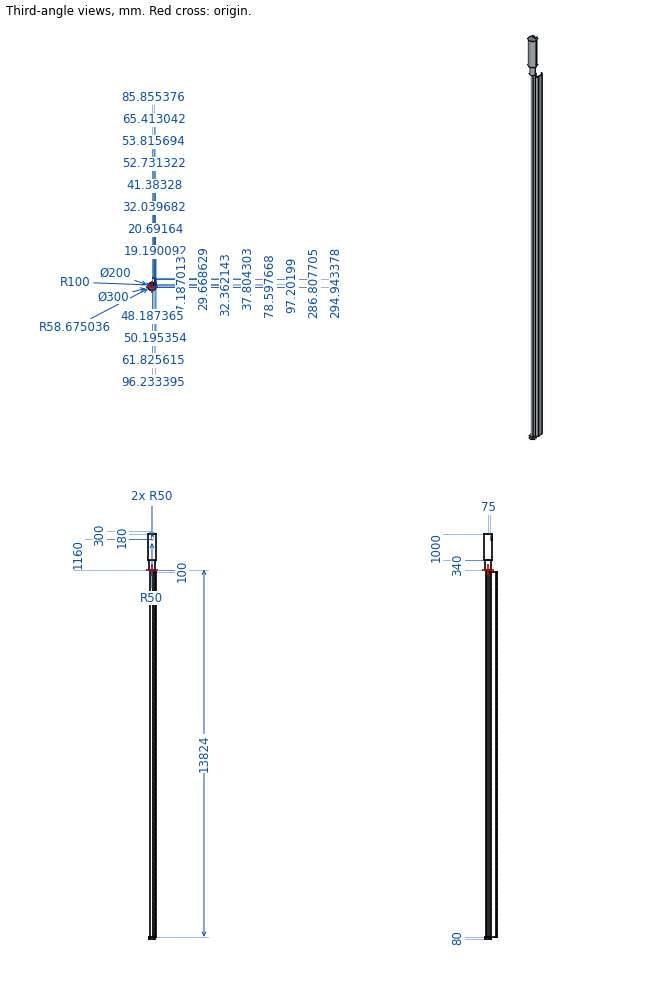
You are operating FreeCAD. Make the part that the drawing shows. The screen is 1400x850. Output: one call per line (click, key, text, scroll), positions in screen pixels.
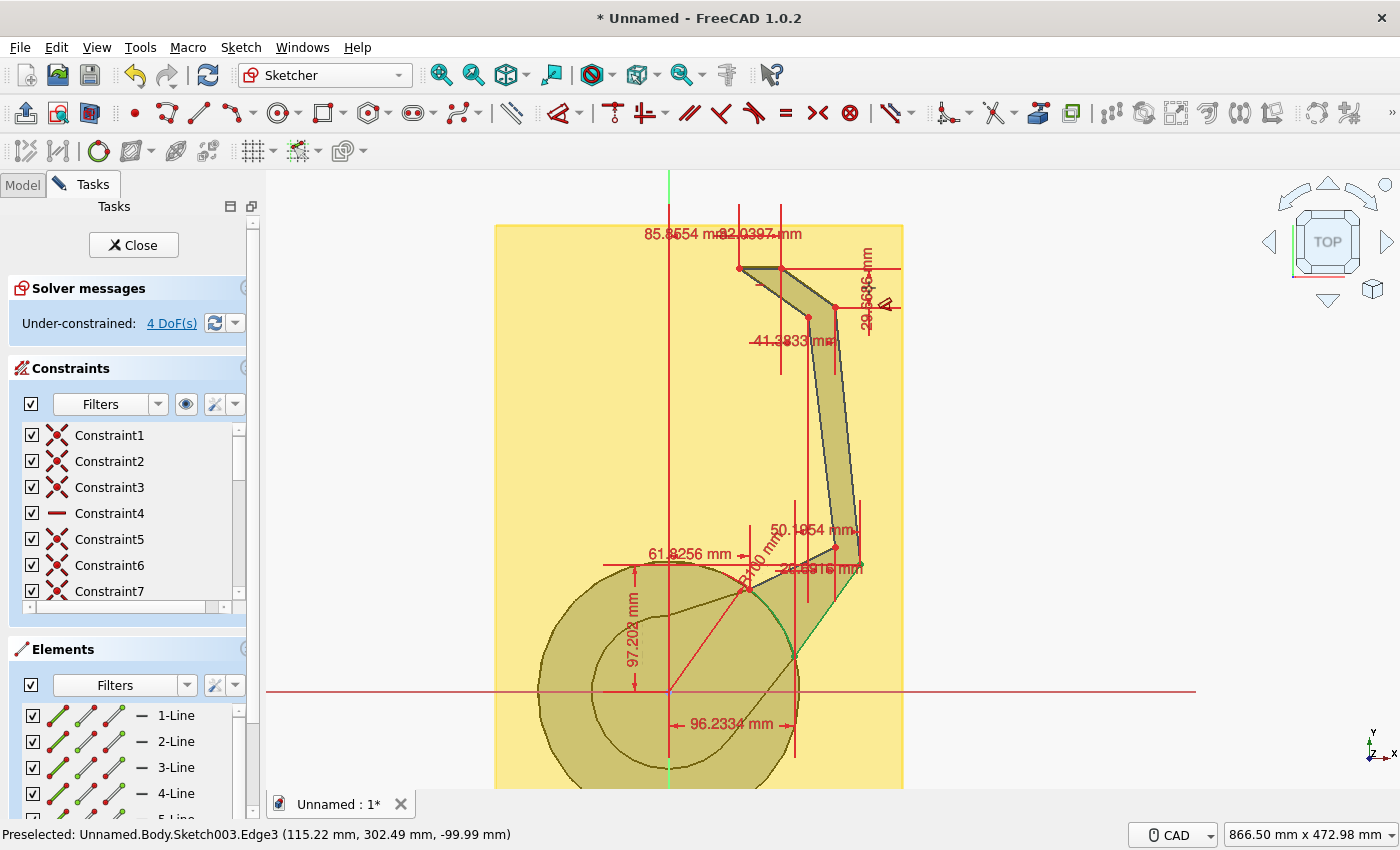
click(760, 283)
click(774, 211)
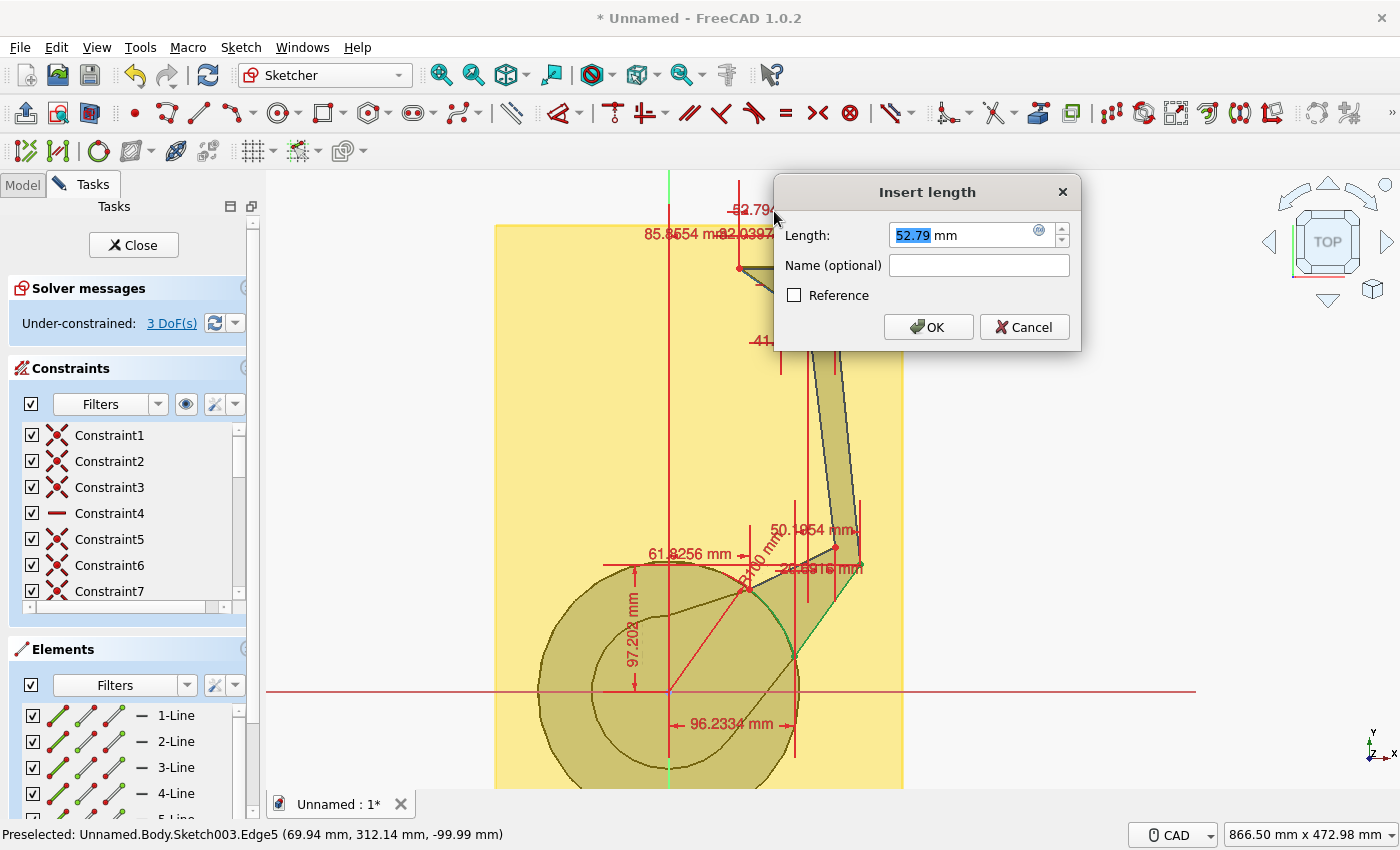
text(52.731322)
key(Return)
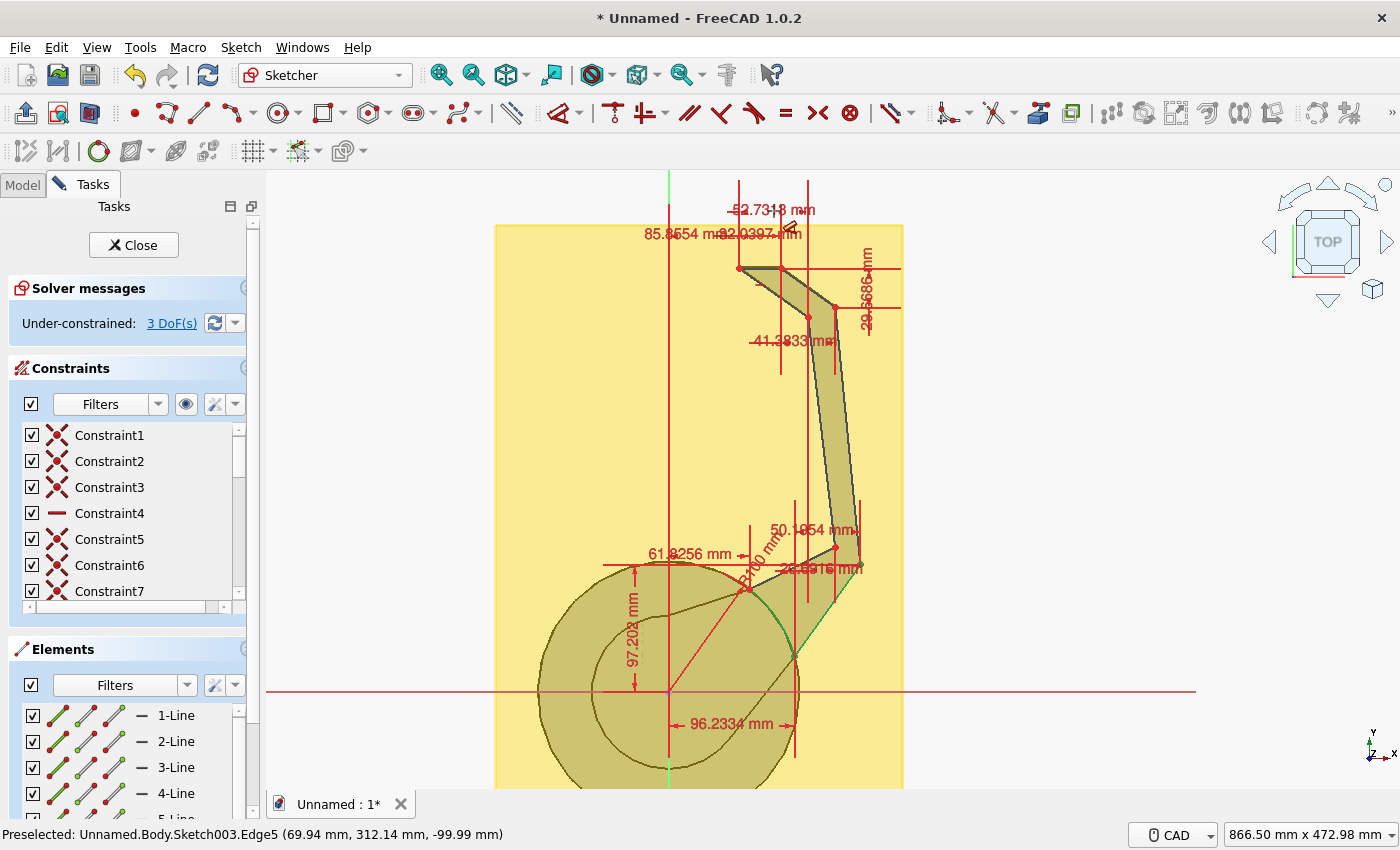
click(760, 283)
click(705, 293)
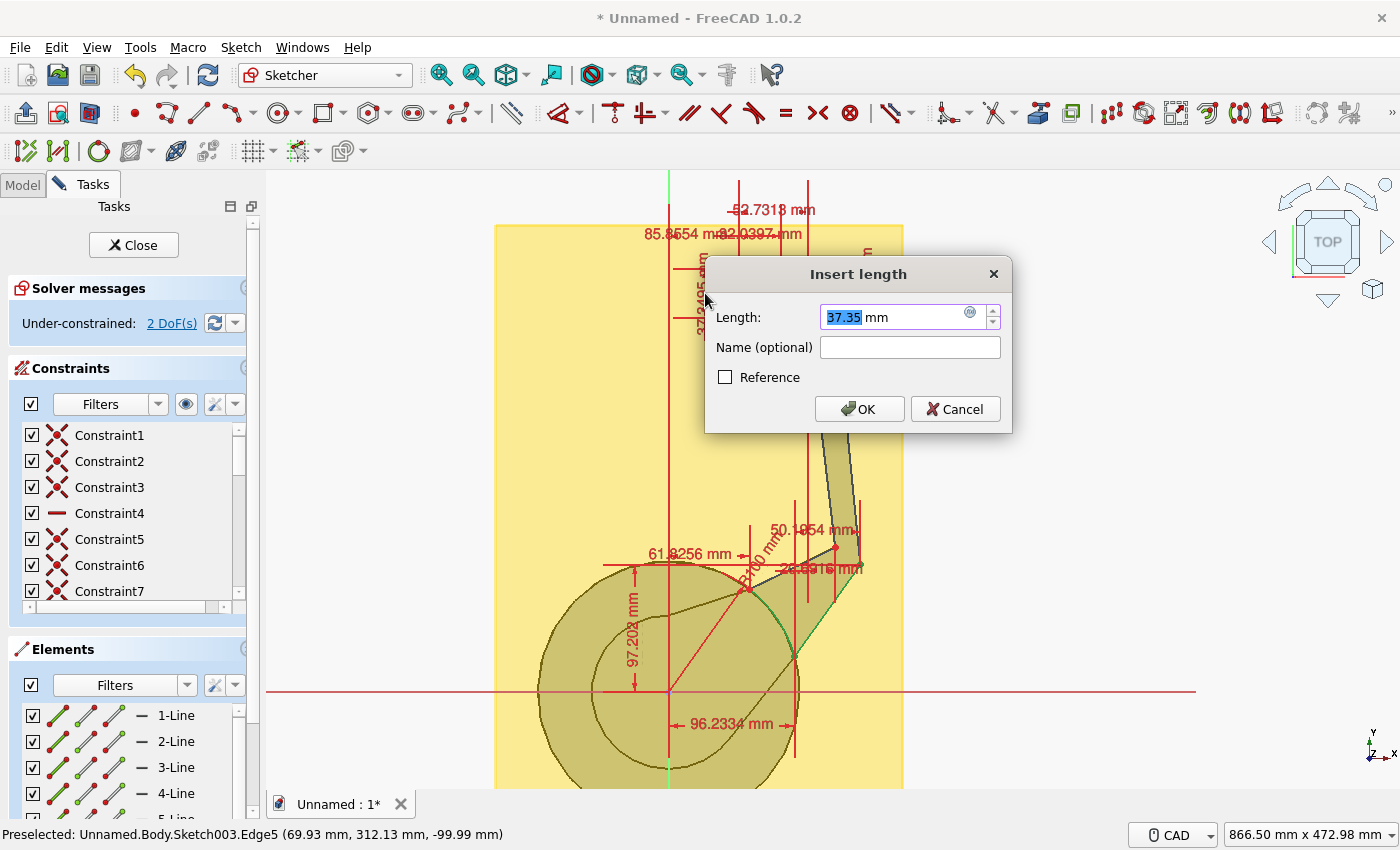
text(37.804303)
key(Return)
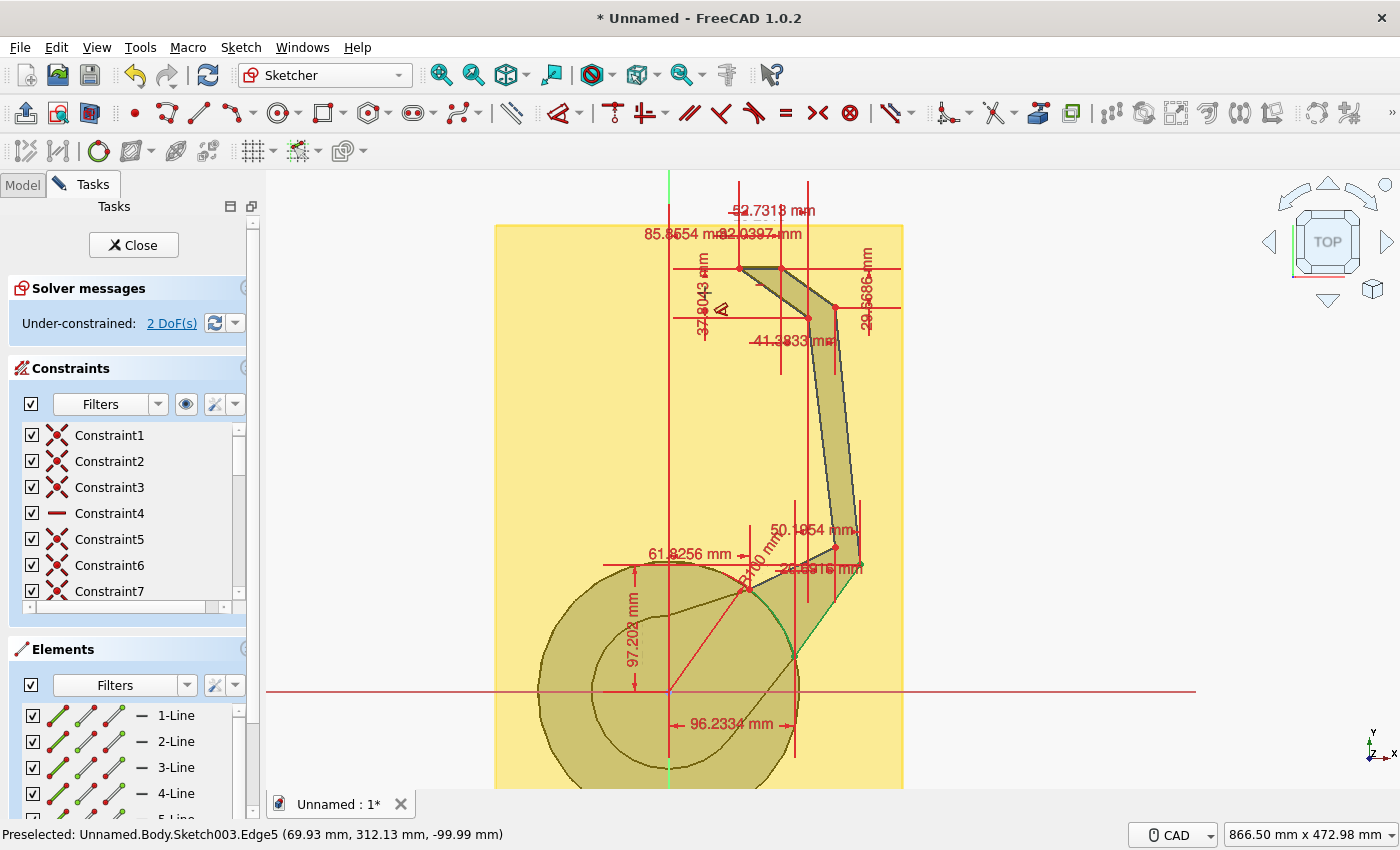
click(810, 560)
click(716, 583)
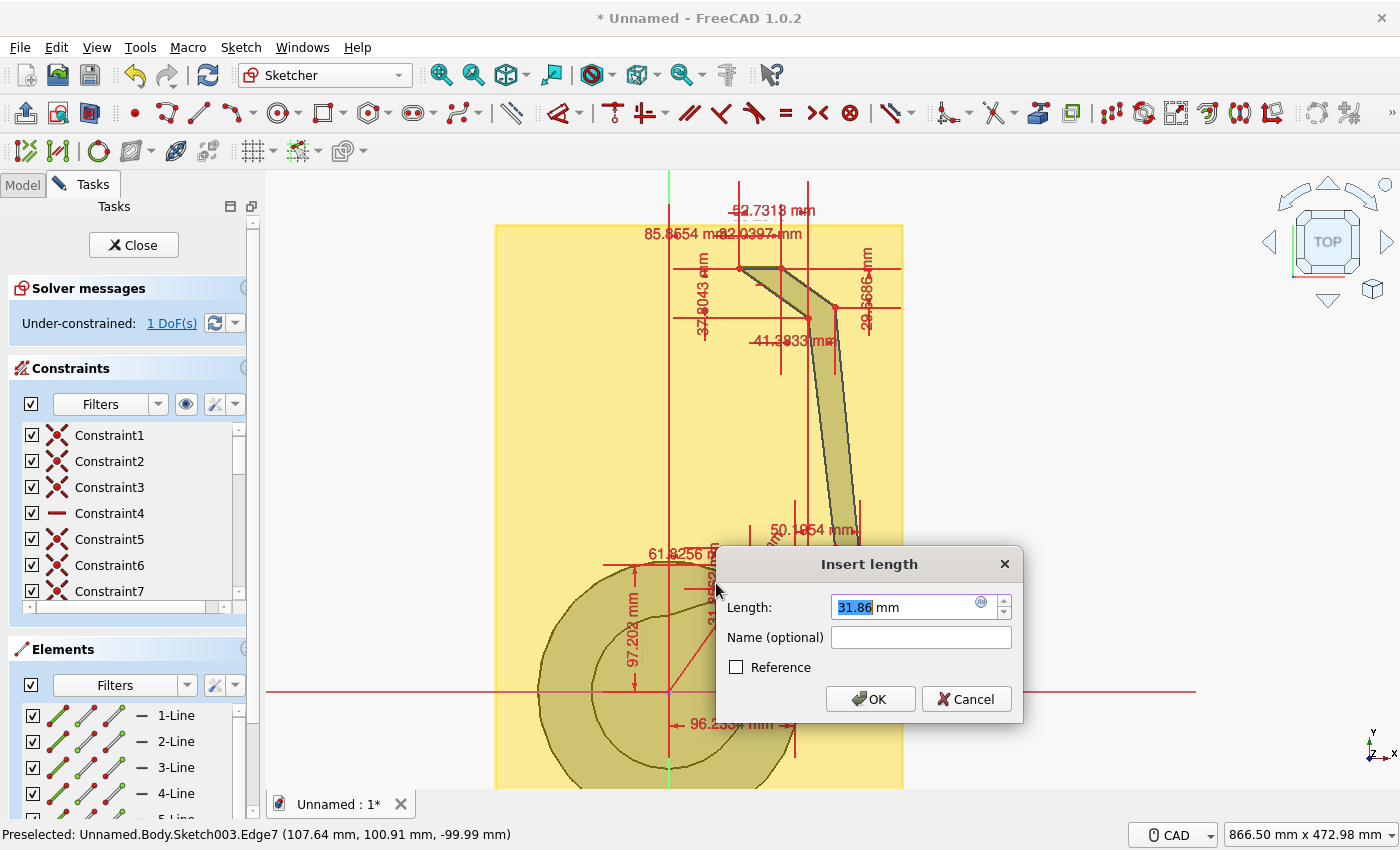
text(32.362143)
key(Return)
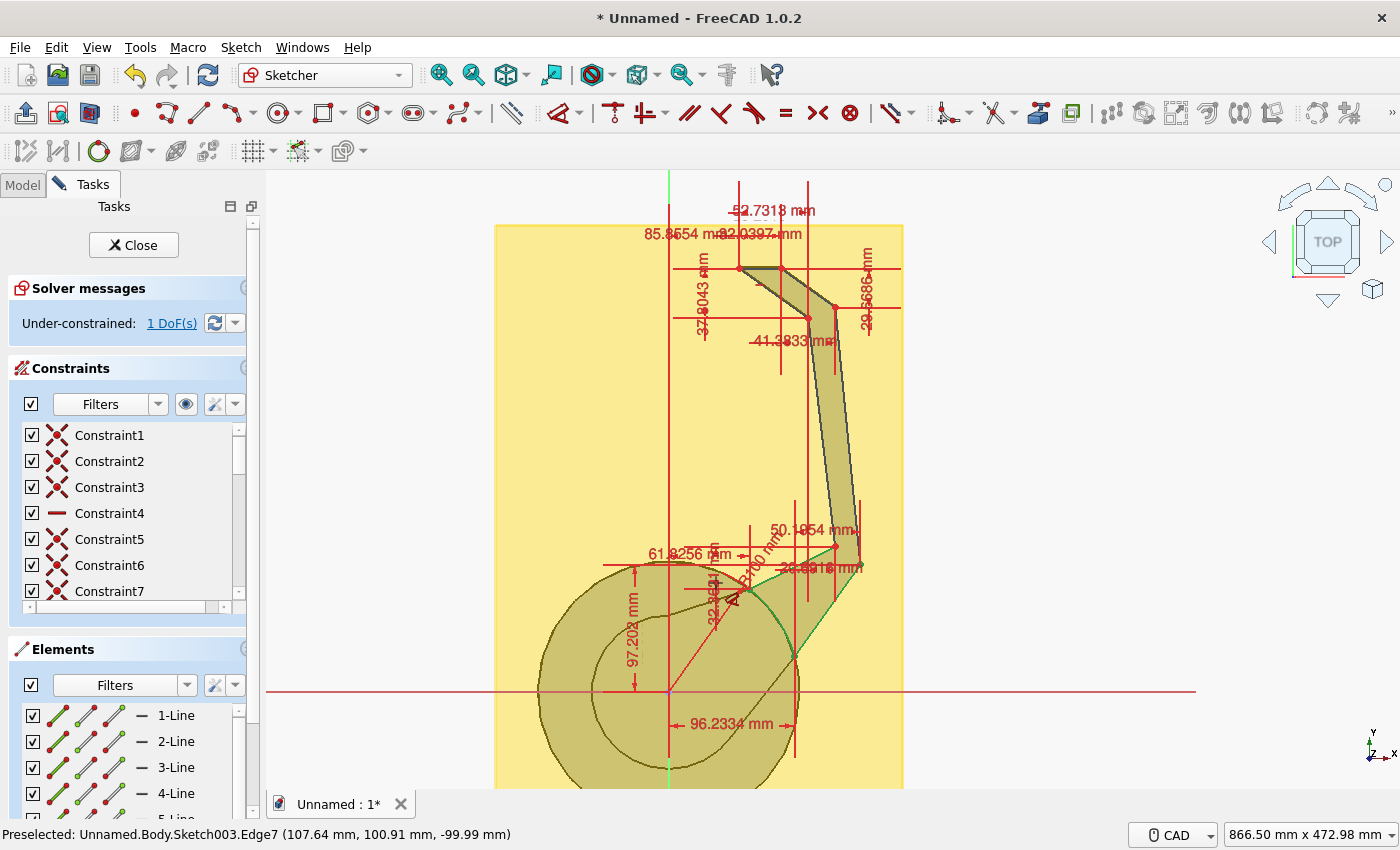
click(835, 308)
click(635, 500)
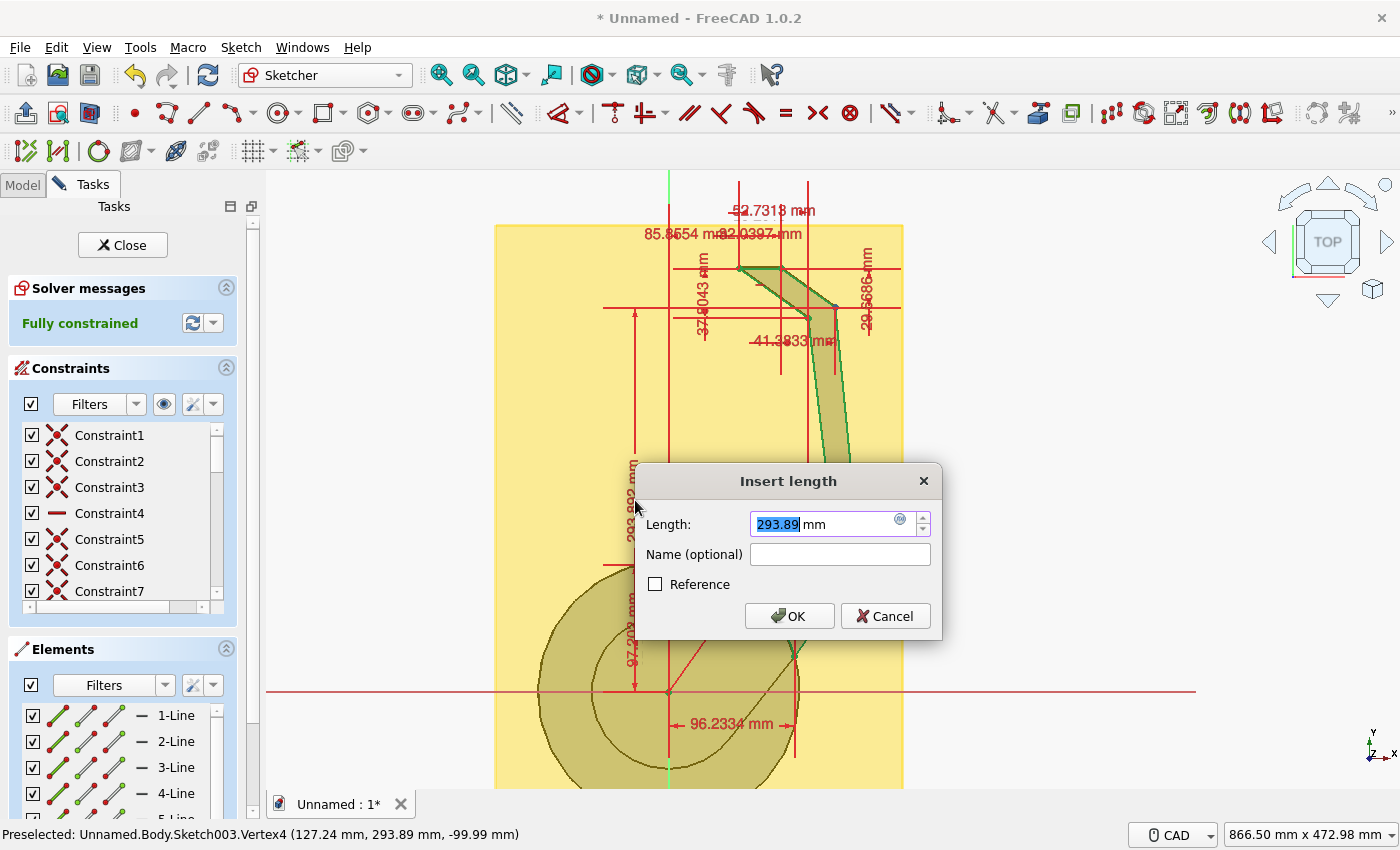
text(294.943378)
key(Return)
key(Escape)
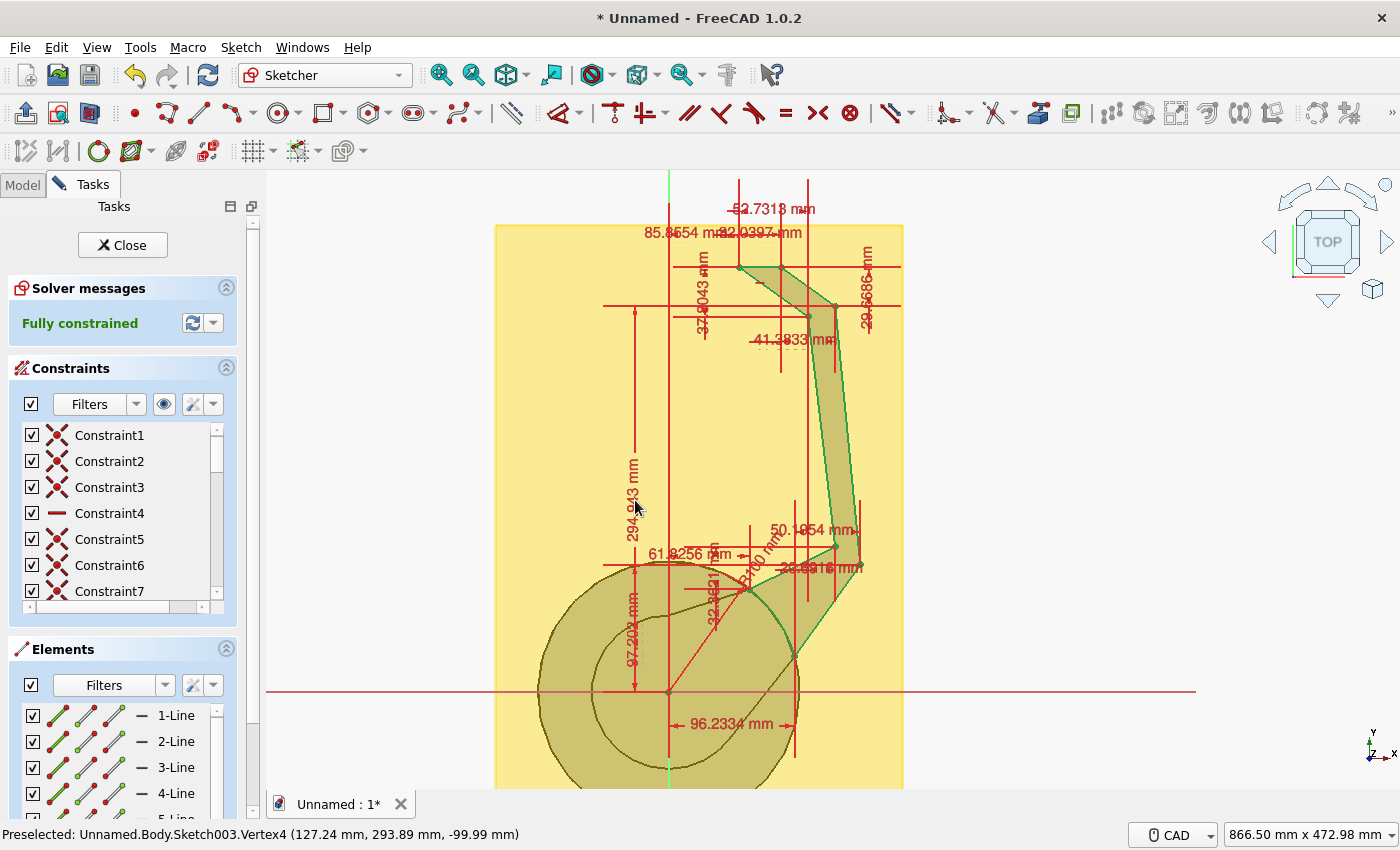
click(123, 245)